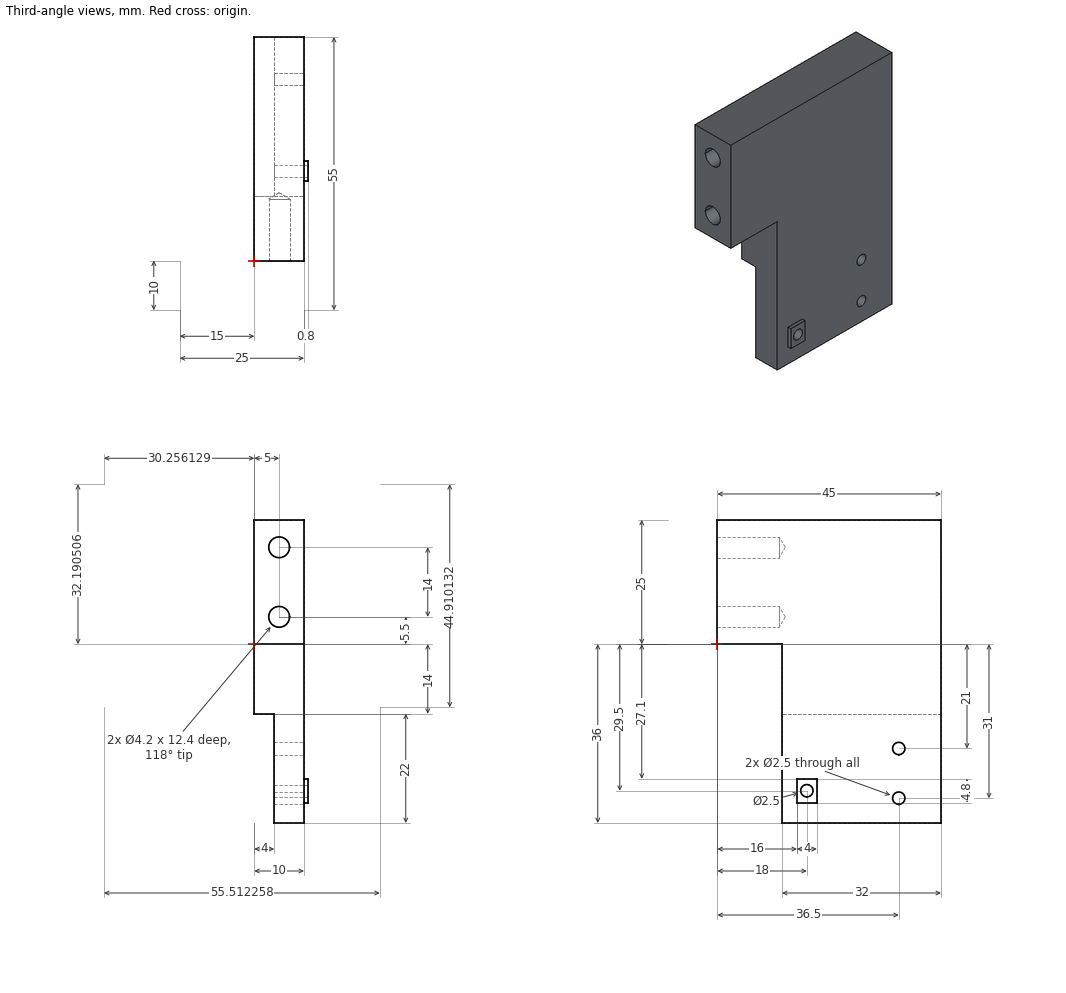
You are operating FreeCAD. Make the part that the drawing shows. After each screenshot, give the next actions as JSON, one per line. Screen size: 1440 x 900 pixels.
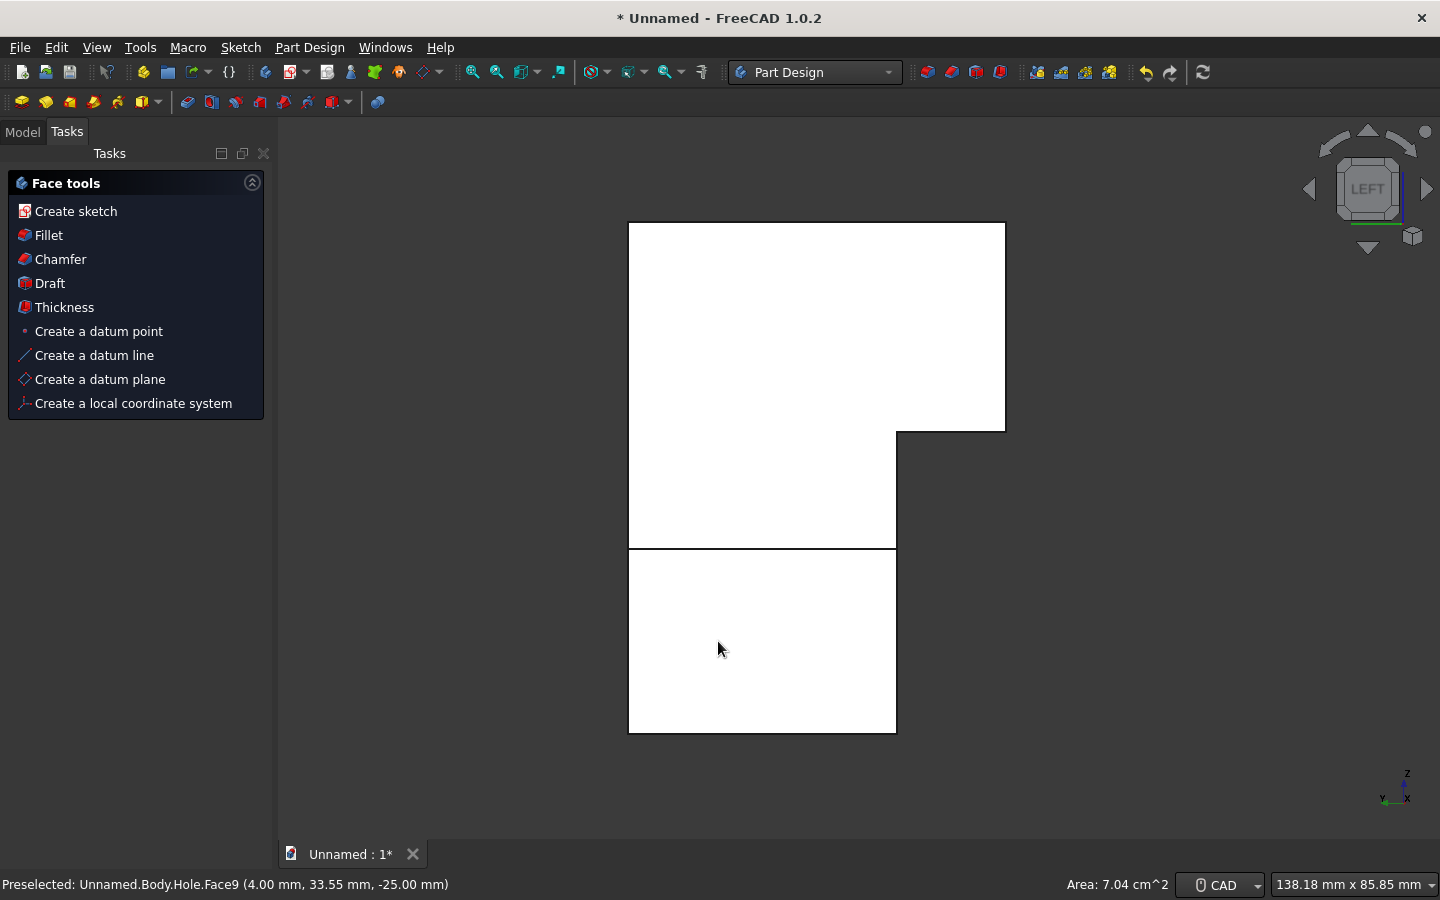
{"action": "left_click", "coordinate": [290, 72]}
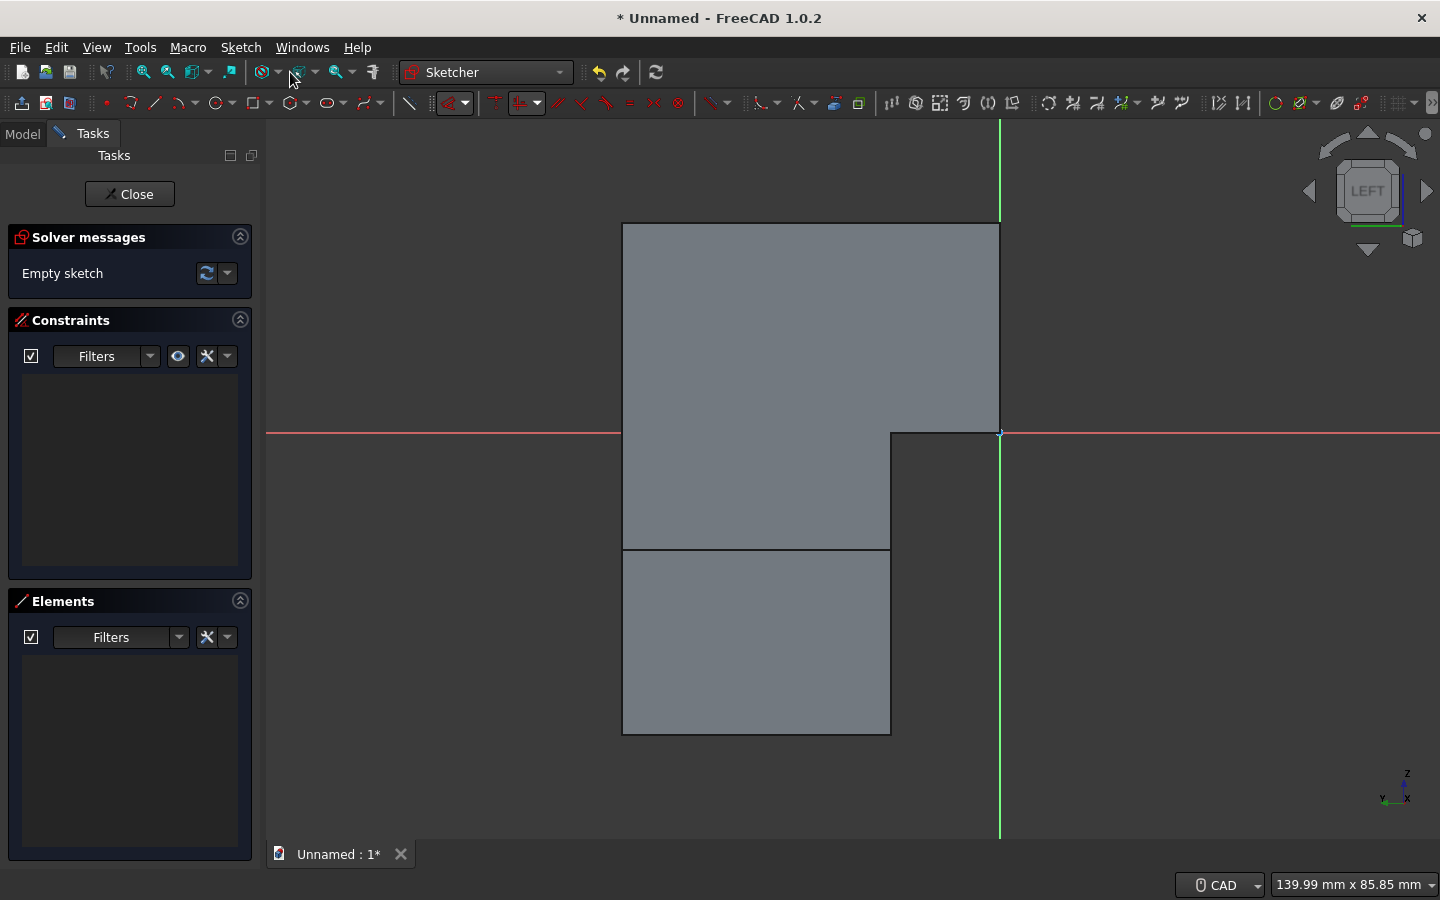
{"action": "left_click", "coordinate": [70, 104]}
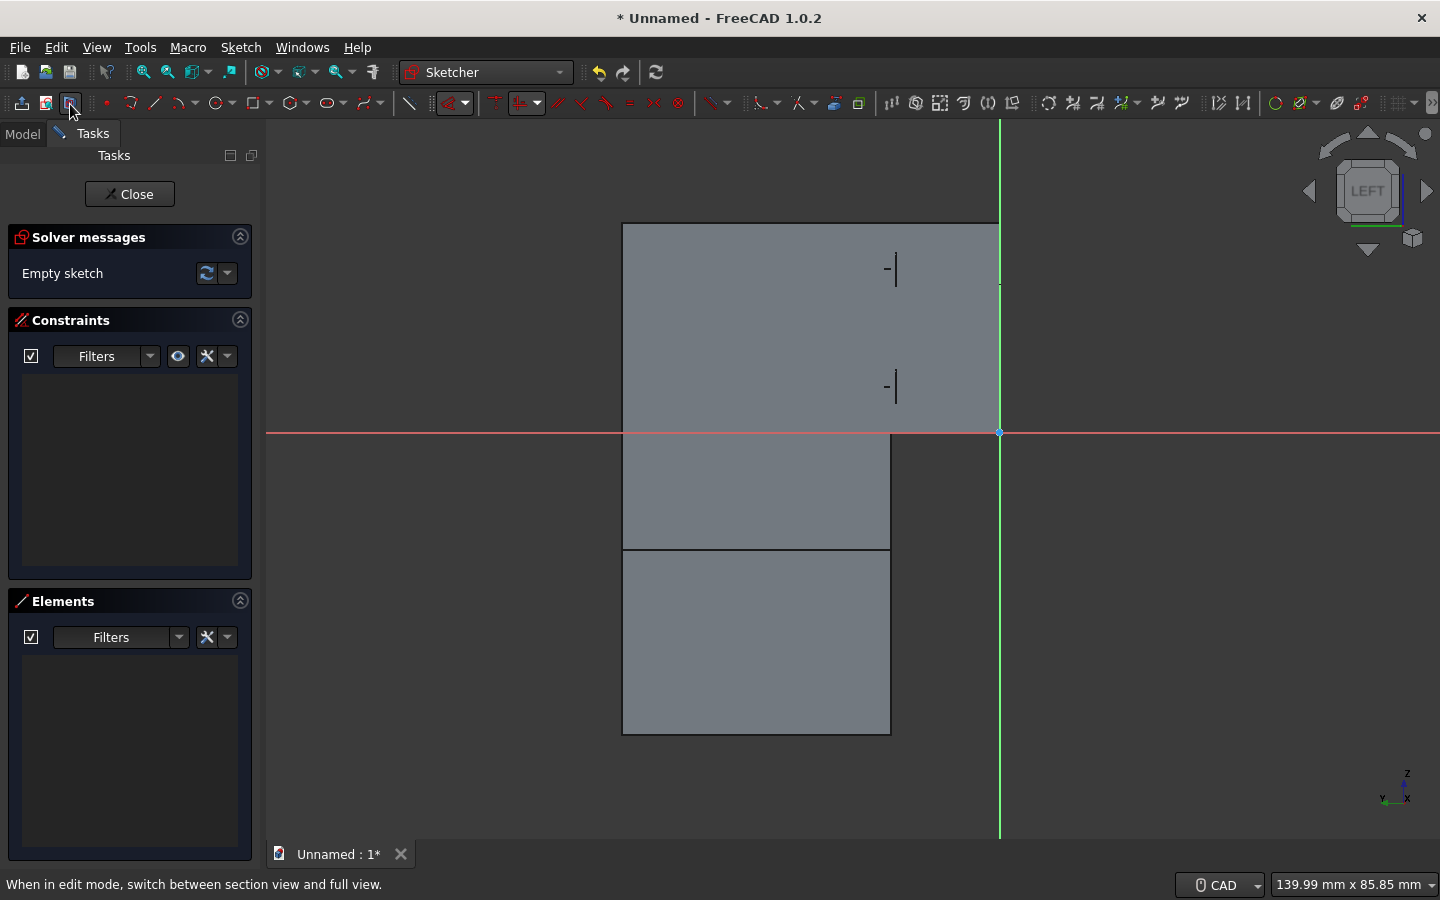
{"action": "scroll", "coordinate": [664, 707], "scroll_direction": "up", "scroll_amount": 7}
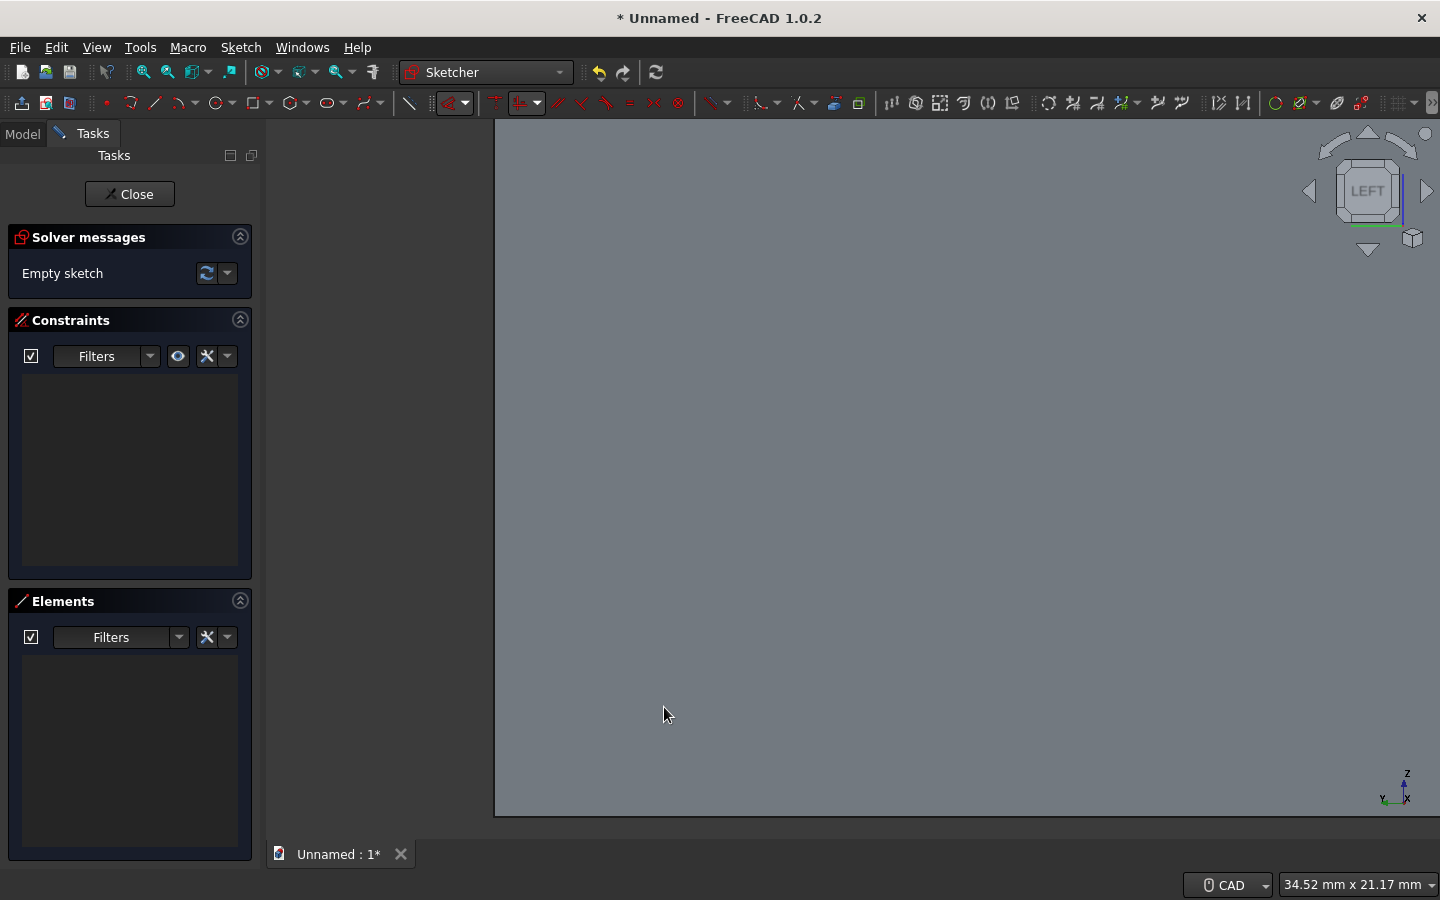
{"action": "left_click", "coordinate": [216, 104]}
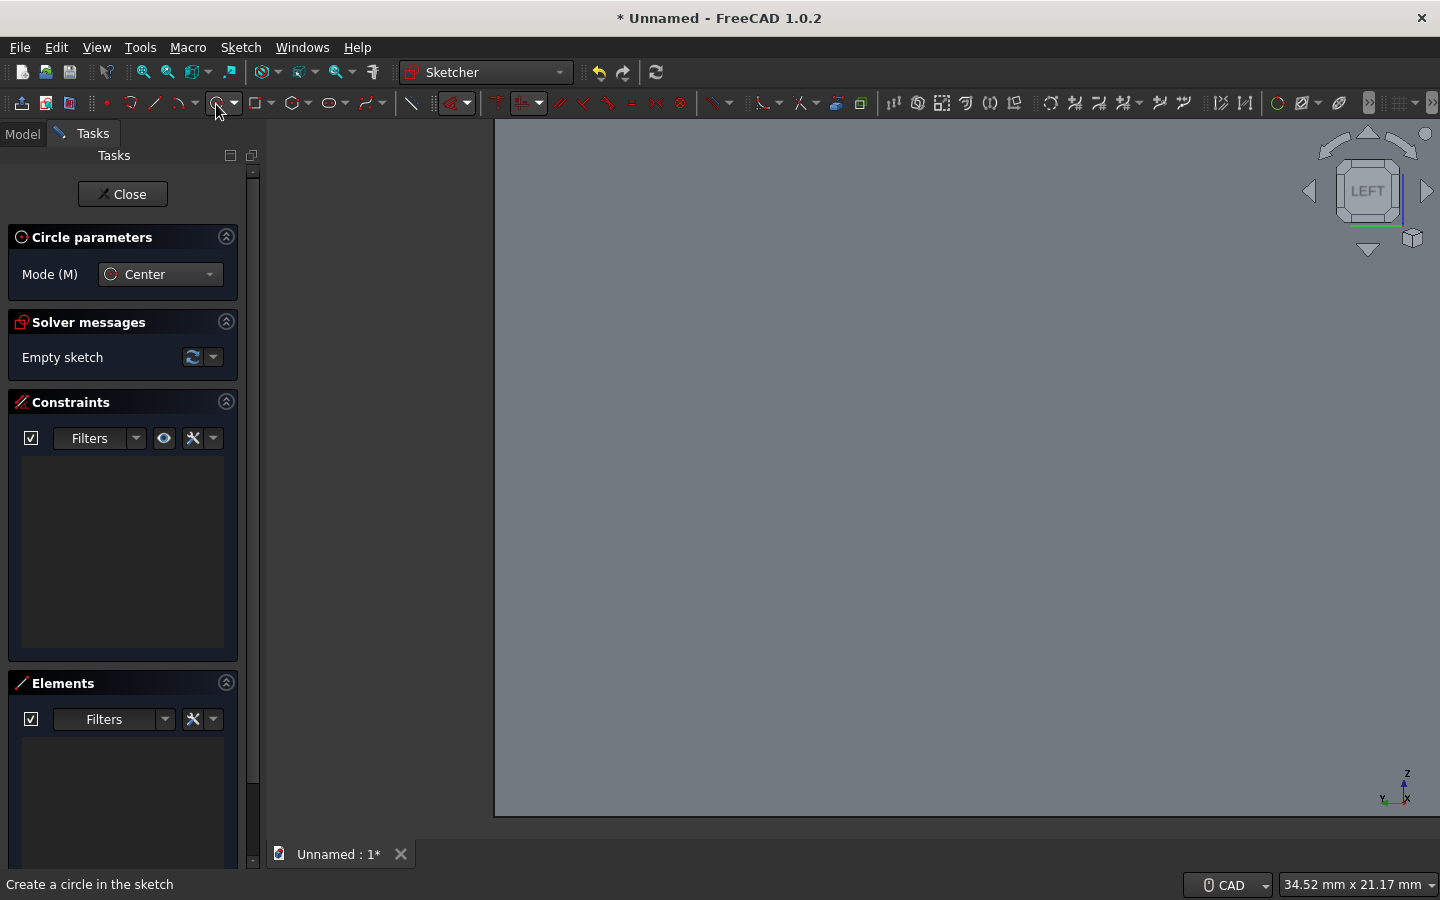
{"action": "left_click", "coordinate": [783, 647]}
{"action": "mouse_move", "coordinate": [813, 617]}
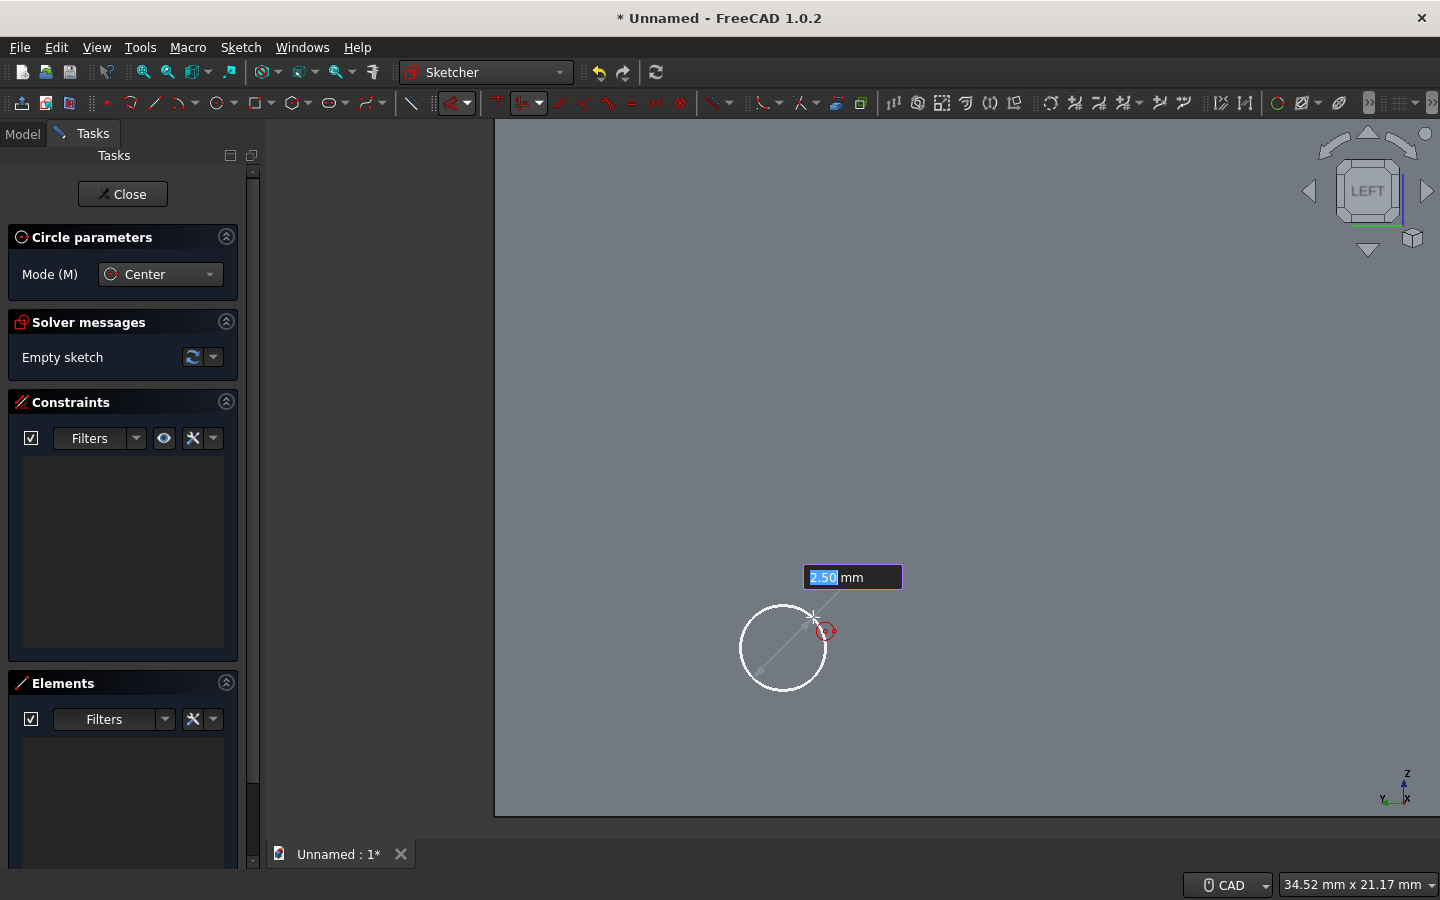
{"action": "type", "text": "2.5"}
{"action": "key", "text": "Return"}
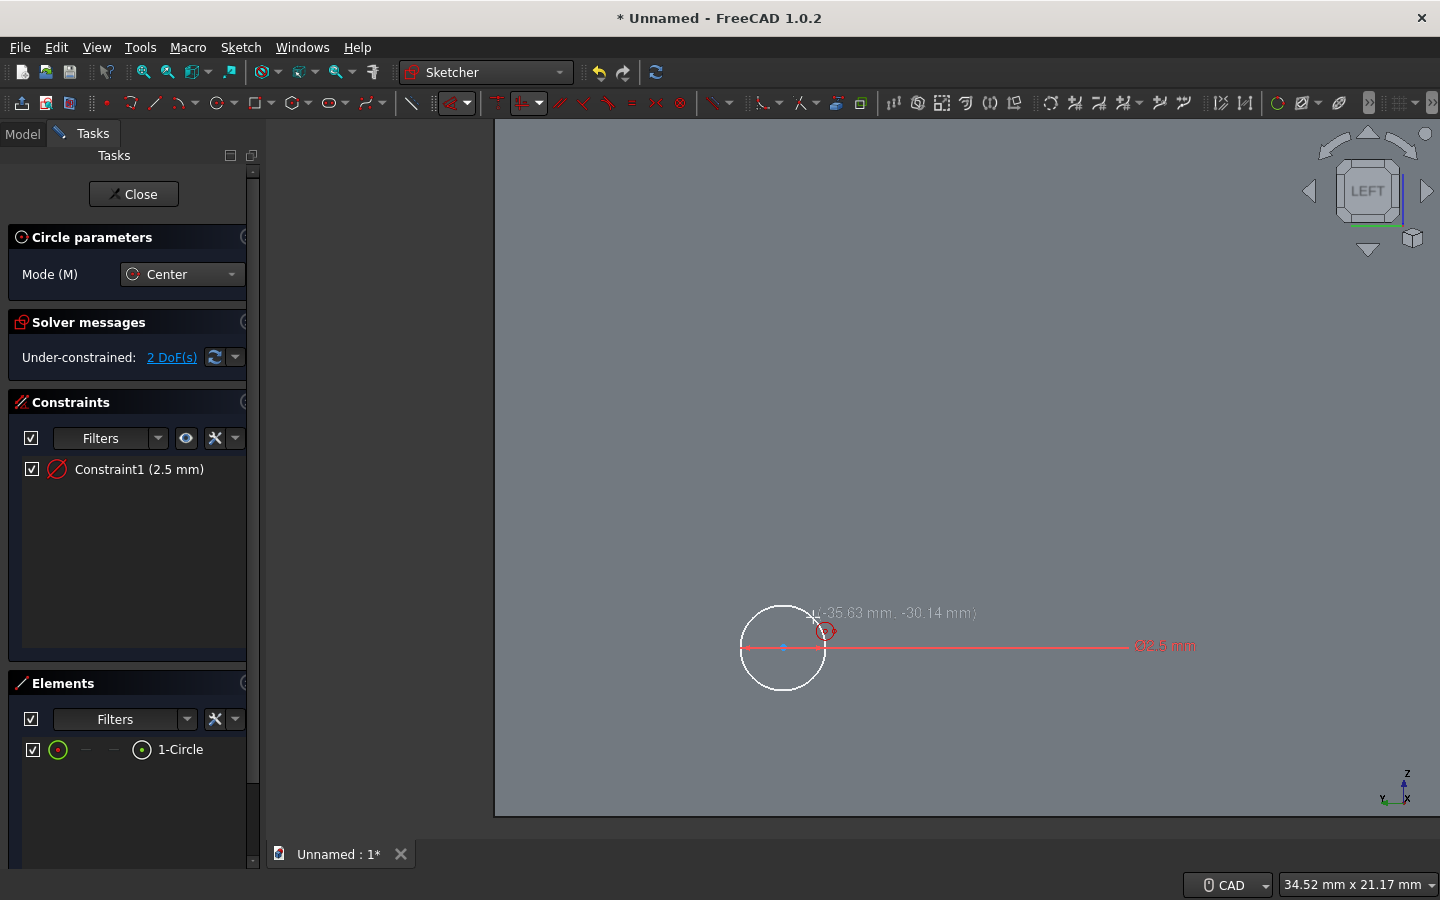
{"action": "left_click", "coordinate": [783, 307]}
{"action": "mouse_move", "coordinate": [813, 277]}